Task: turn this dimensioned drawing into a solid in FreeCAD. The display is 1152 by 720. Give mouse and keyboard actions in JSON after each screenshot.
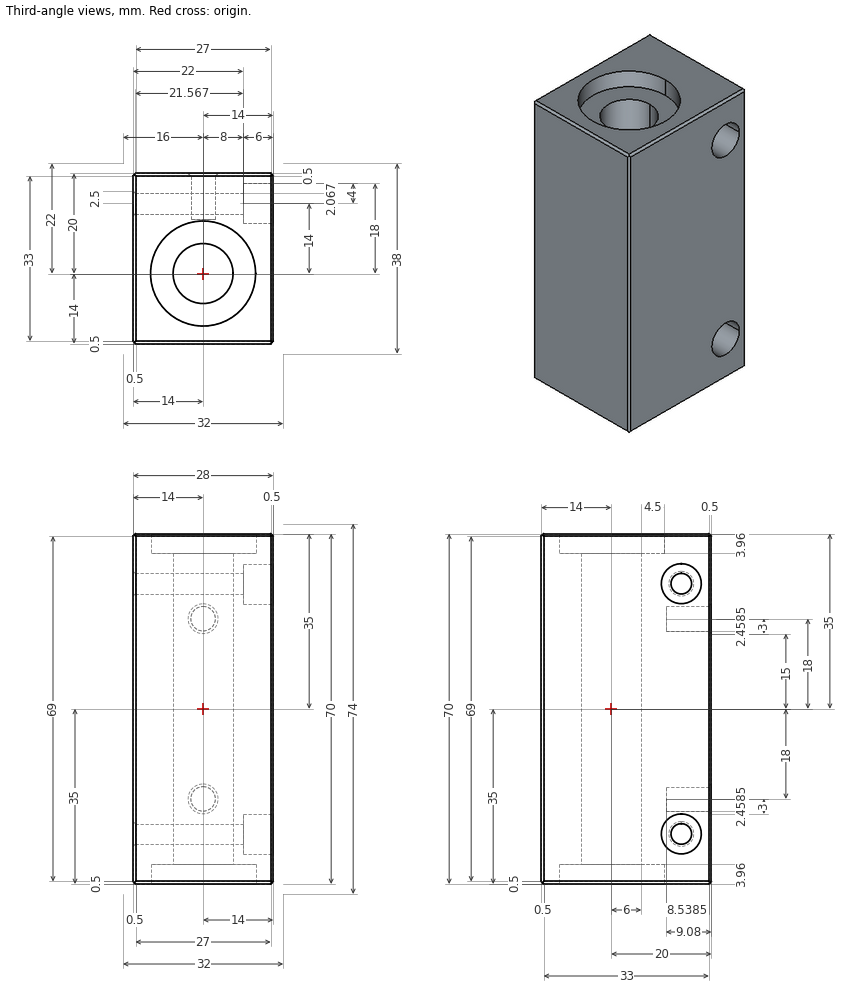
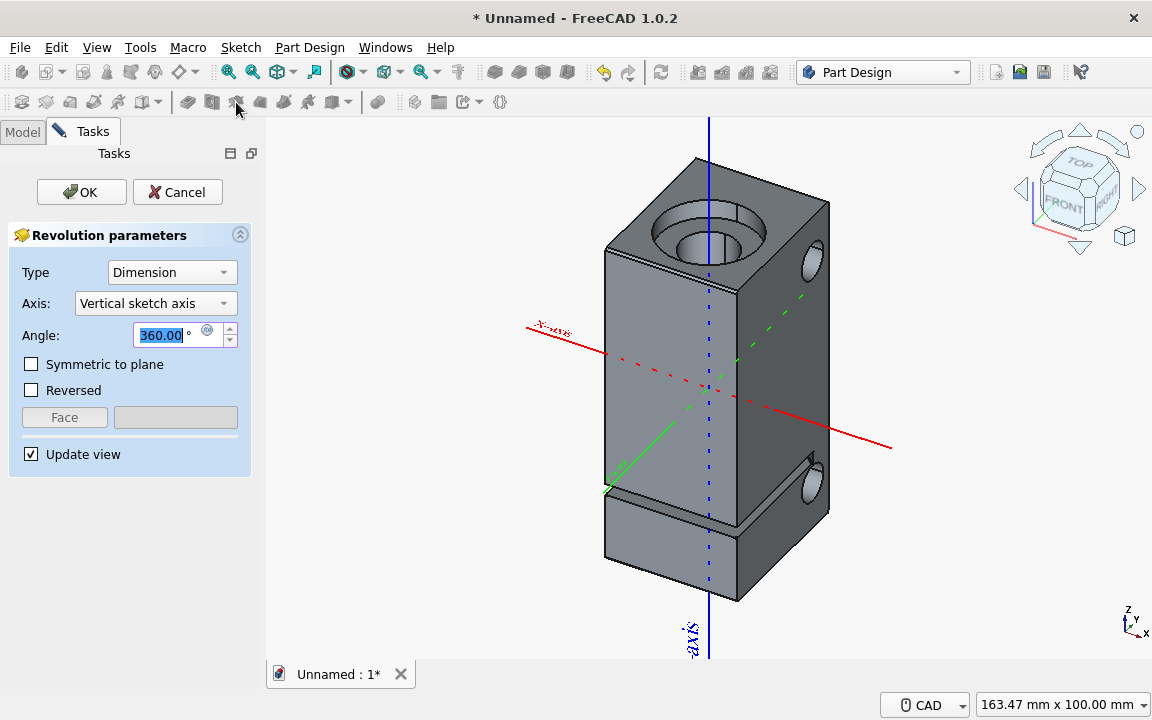
{"action": "left_click", "coordinate": [156, 304]}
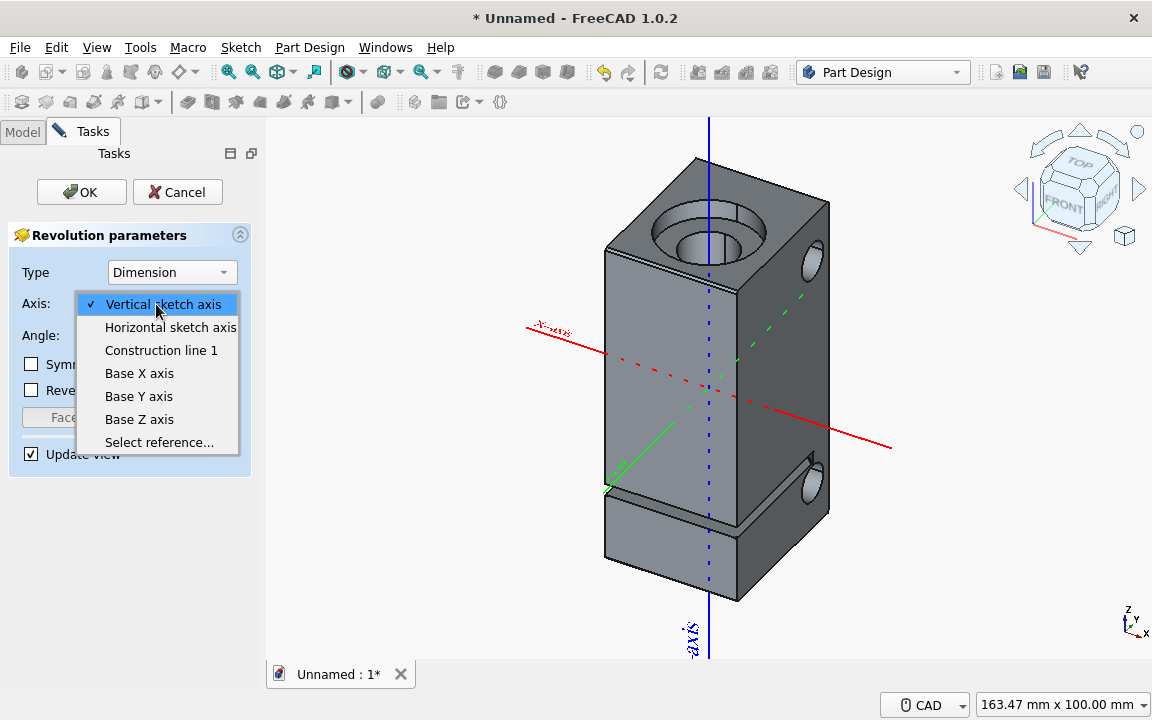
{"action": "left_click", "coordinate": [156, 350]}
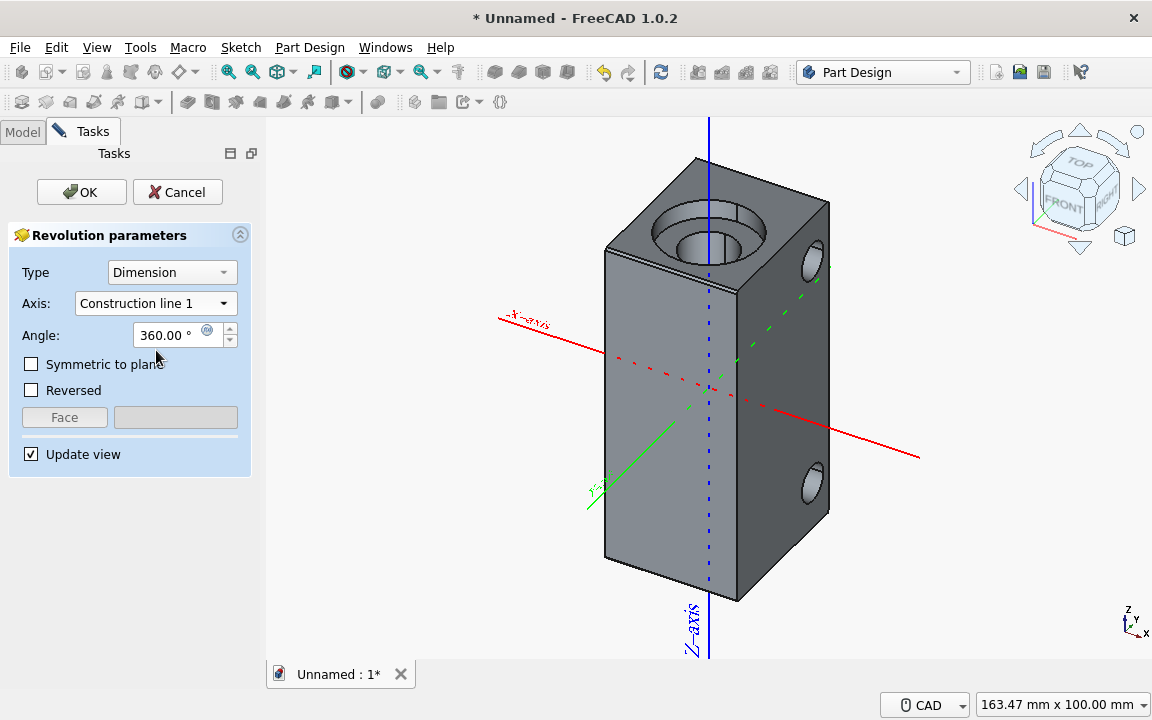
{"action": "left_click", "coordinate": [82, 192]}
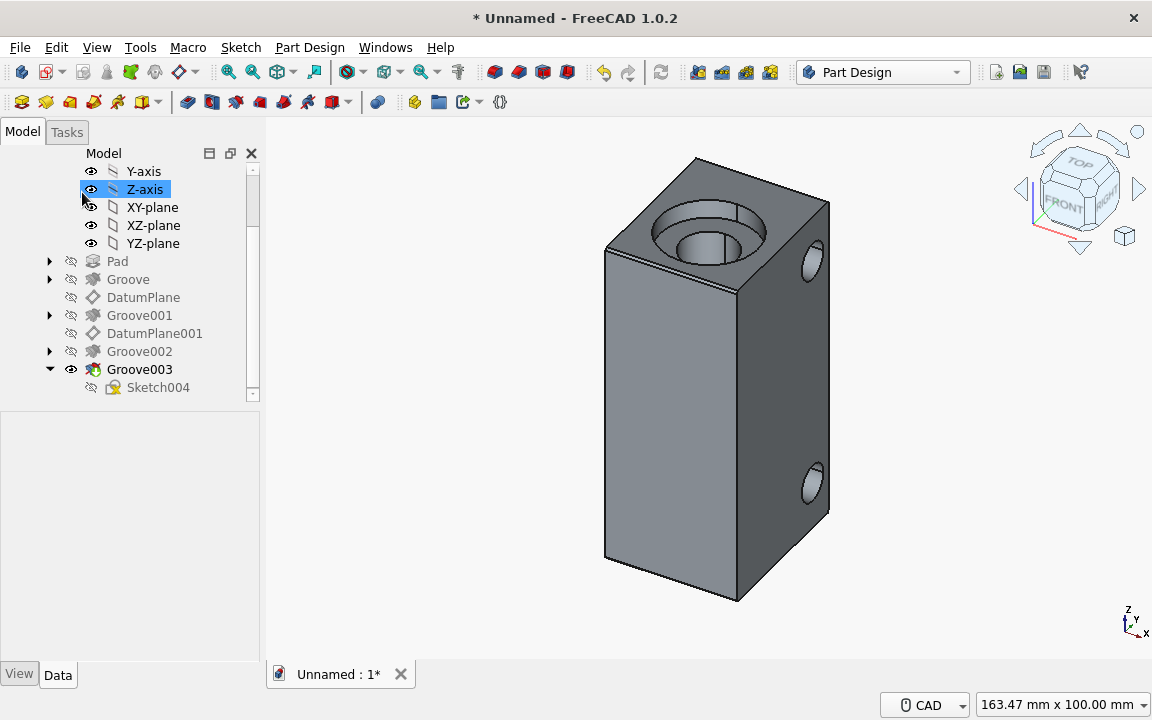
{"action": "left_click", "coordinate": [46, 72]}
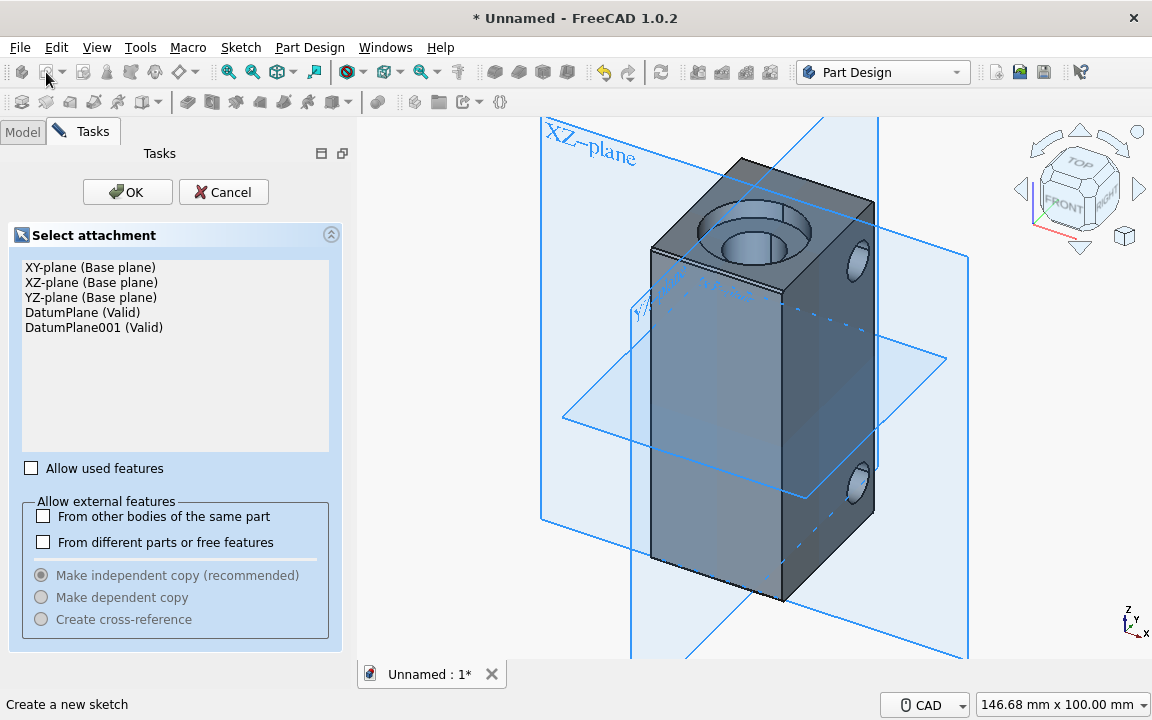
{"action": "left_click", "coordinate": [82, 298]}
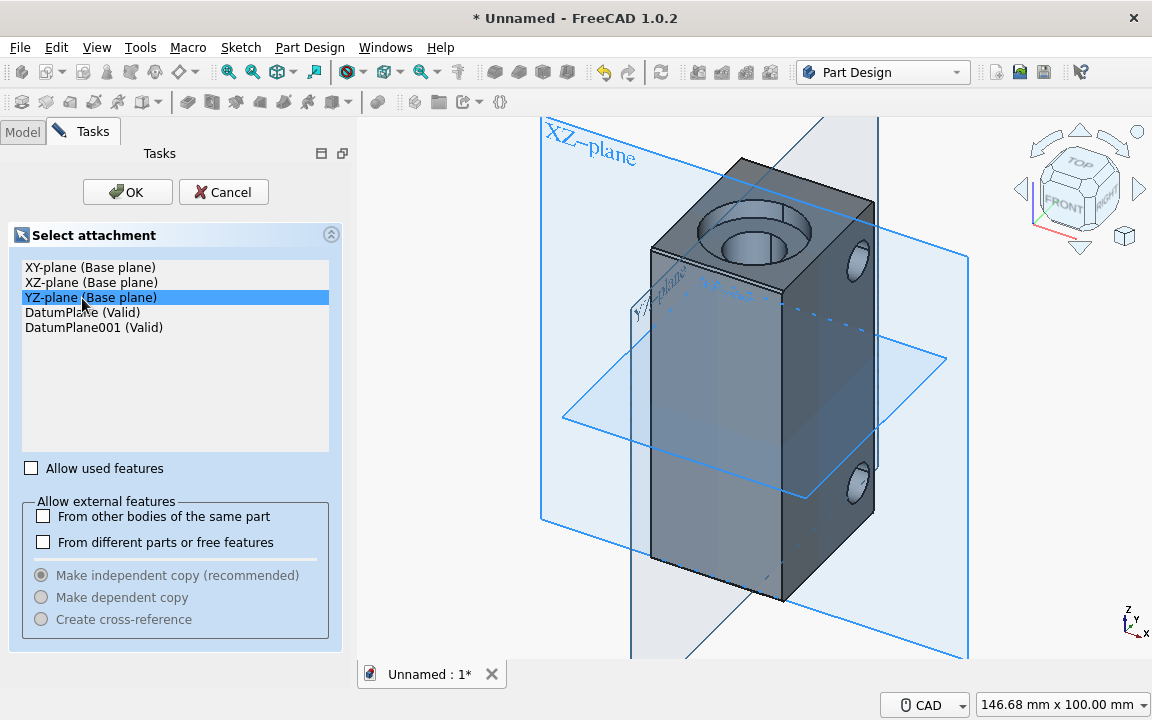
{"action": "left_click", "coordinate": [128, 192]}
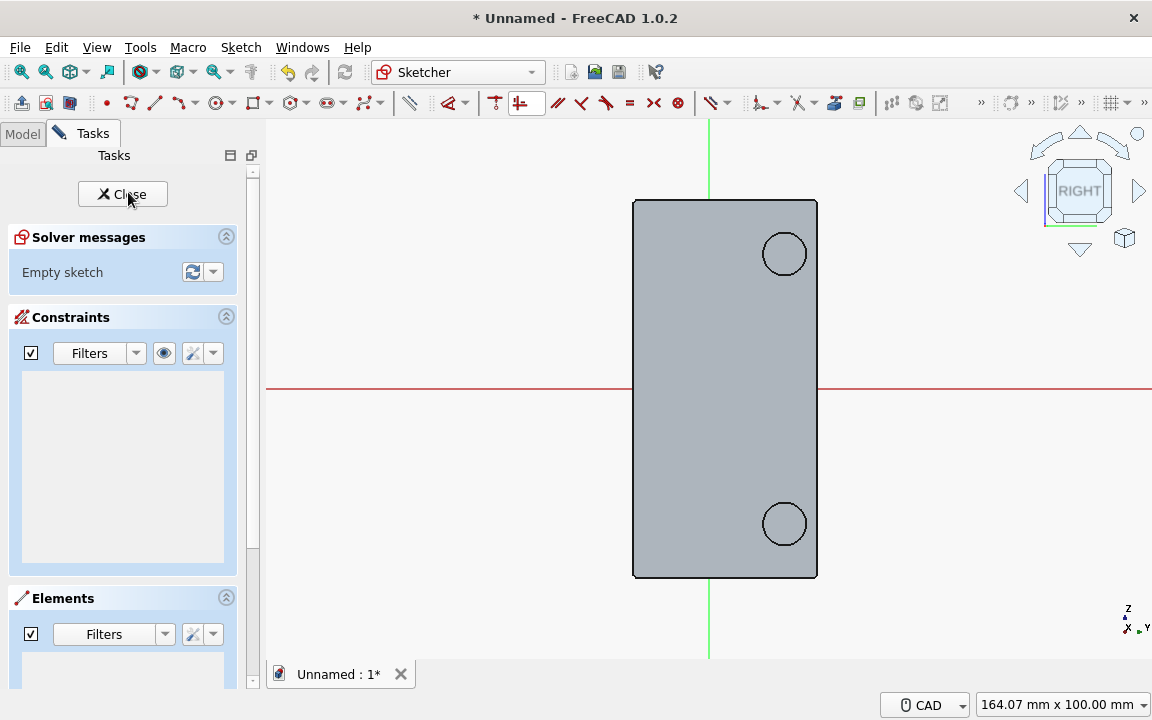
{"action": "key", "text": "q s"}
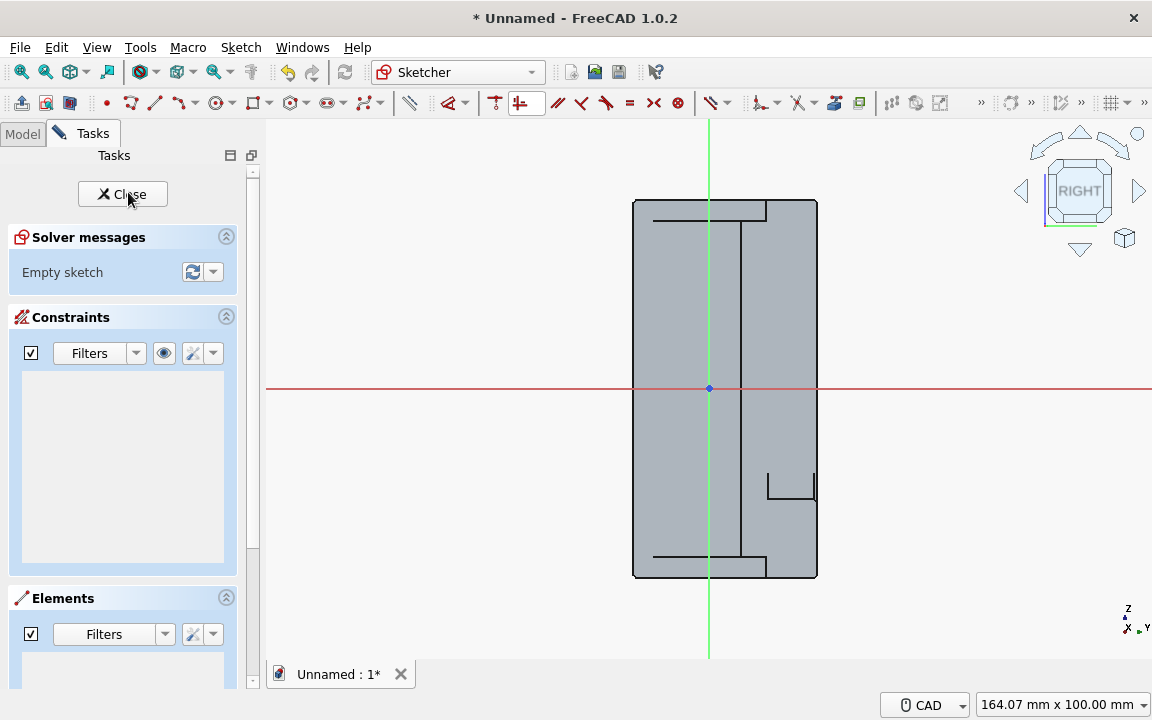
{"action": "scroll", "coordinate": [830, 319], "scroll_direction": "up", "scroll_amount": 6}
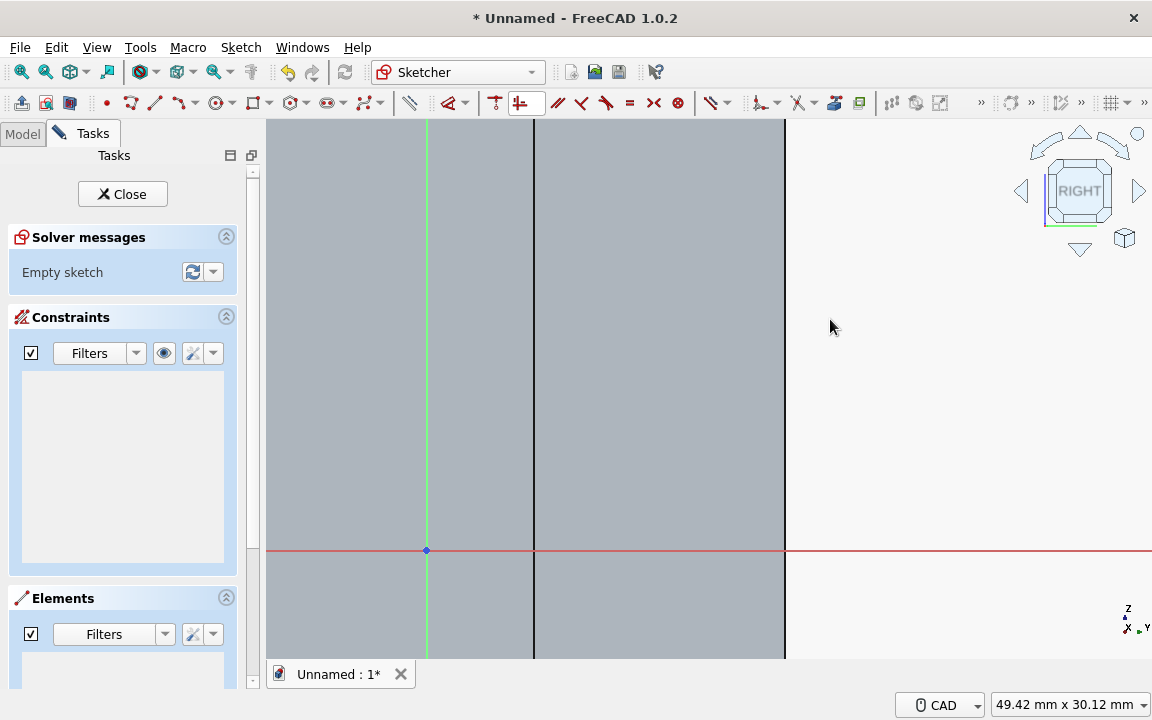
{"action": "left_click", "coordinate": [132, 104]}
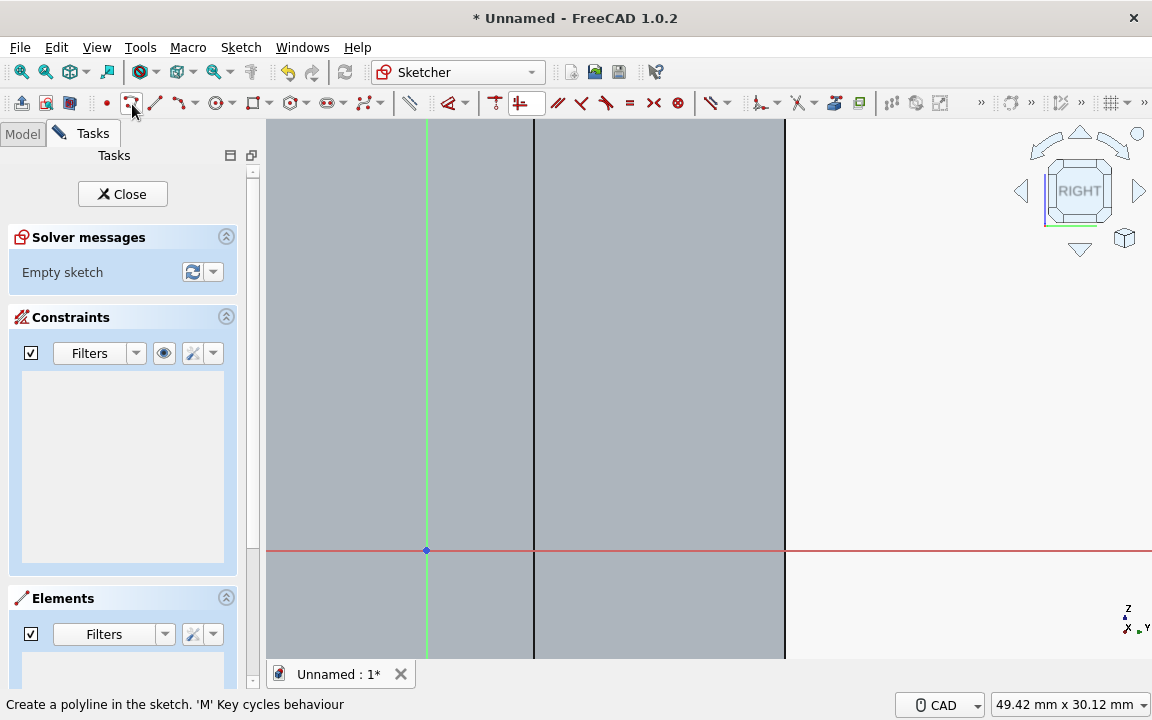
{"action": "left_click", "coordinate": [623, 272]}
{"action": "left_click", "coordinate": [776, 272]}
{"action": "left_click", "coordinate": [785, 282]}
{"action": "left_click", "coordinate": [785, 228]}
{"action": "left_click", "coordinate": [623, 228]}
{"action": "left_click", "coordinate": [623, 273]}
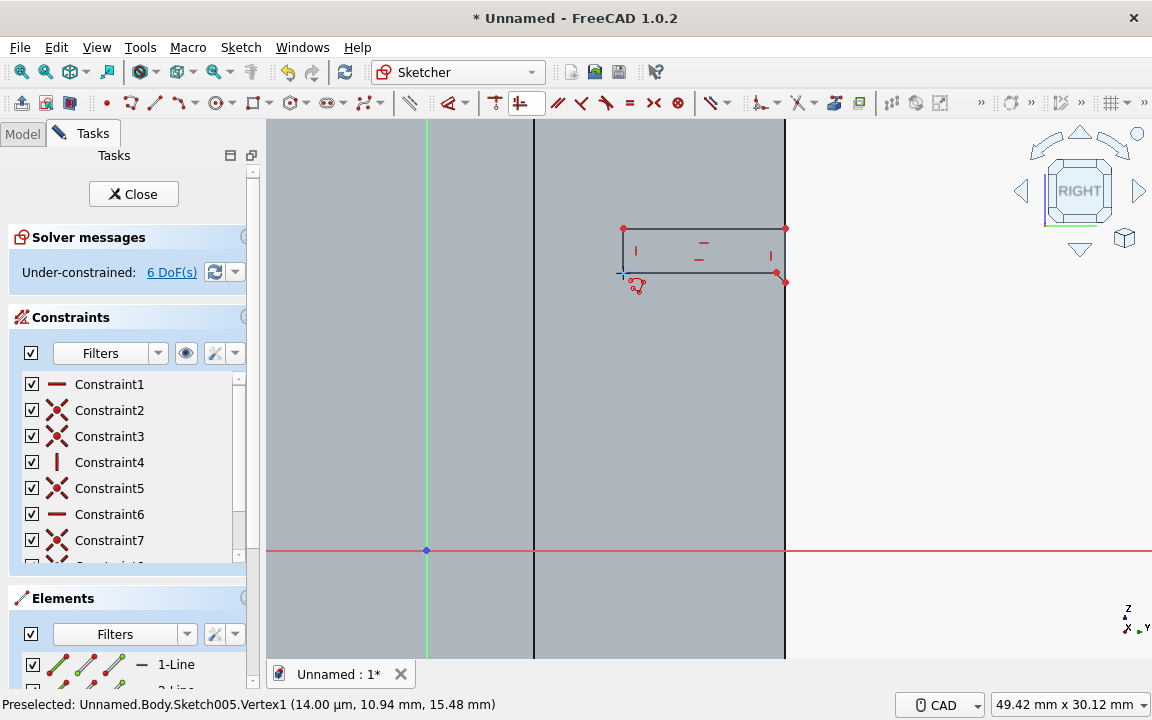
{"action": "left_click", "coordinate": [156, 104]}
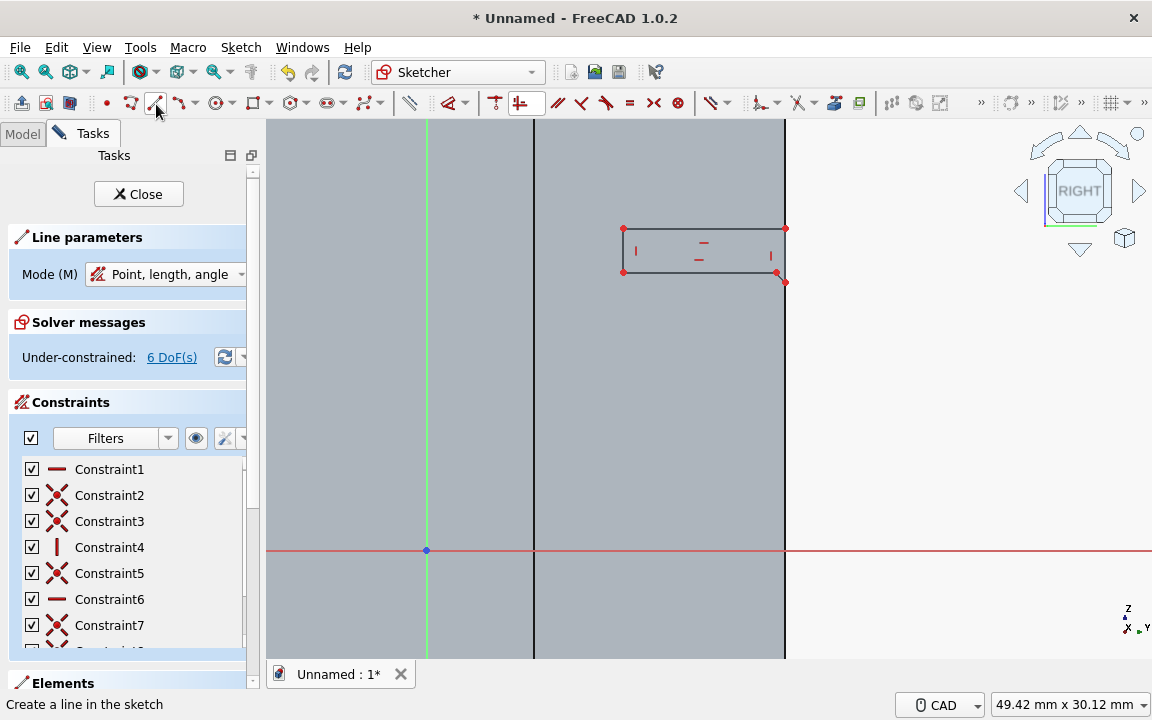
{"action": "left_click", "coordinate": [802, 228]}
{"action": "left_click", "coordinate": [850, 228]}
{"action": "key", "text": "Escape"}